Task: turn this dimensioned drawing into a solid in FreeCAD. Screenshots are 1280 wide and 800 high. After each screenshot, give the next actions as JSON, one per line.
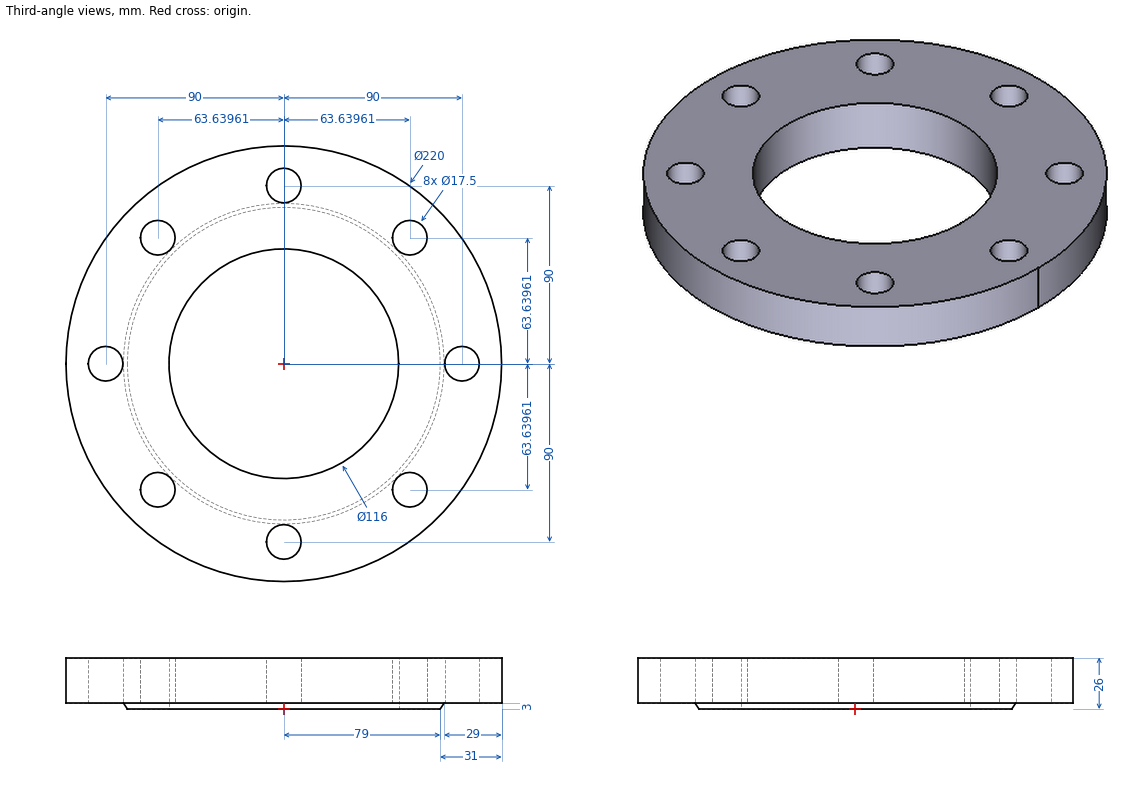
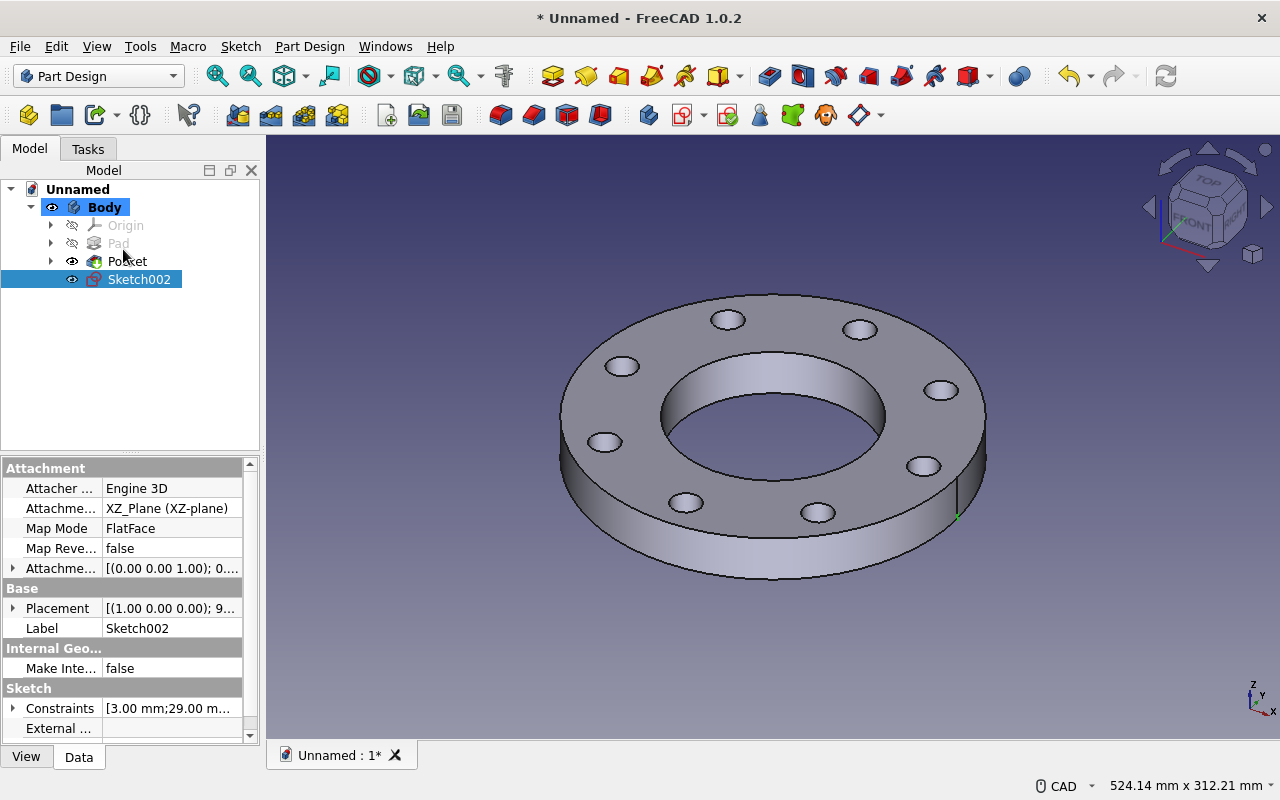
{"action": "left_click", "coordinate": [836, 76]}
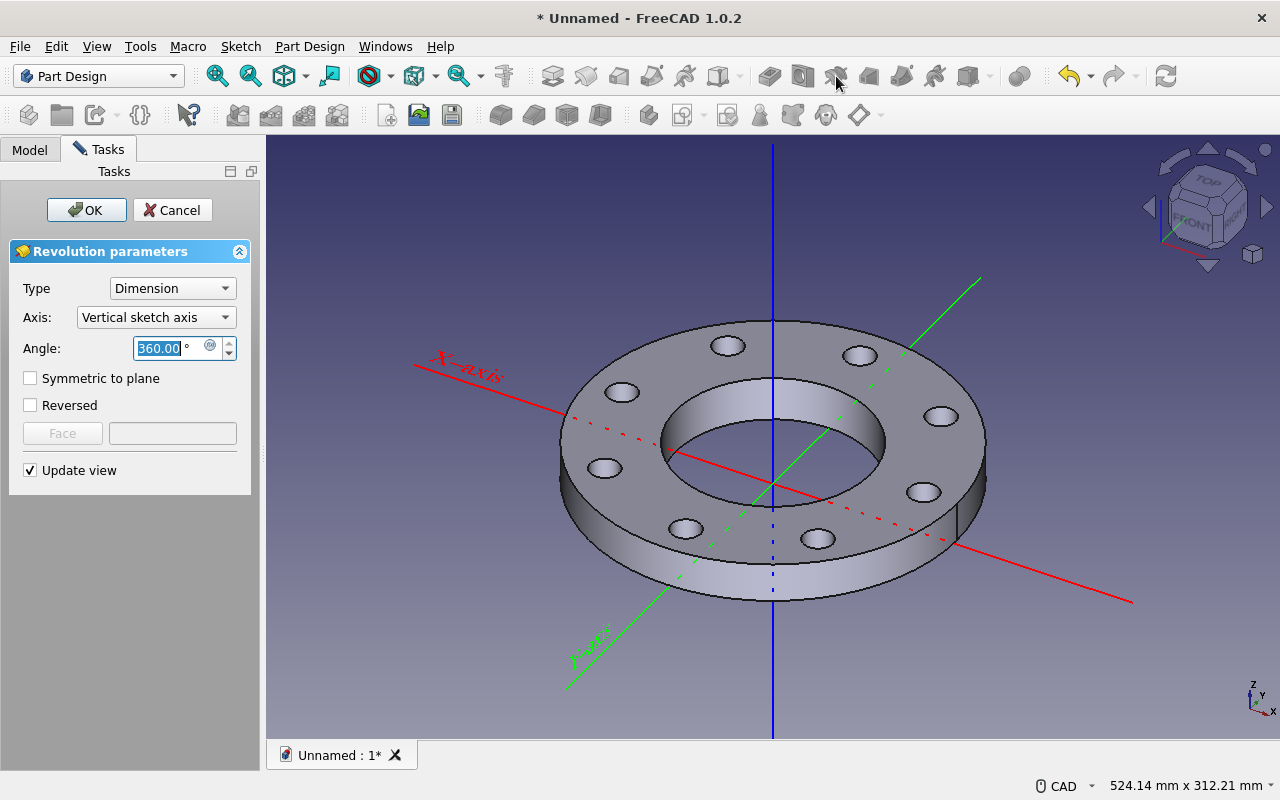
{"action": "left_click", "coordinate": [87, 210]}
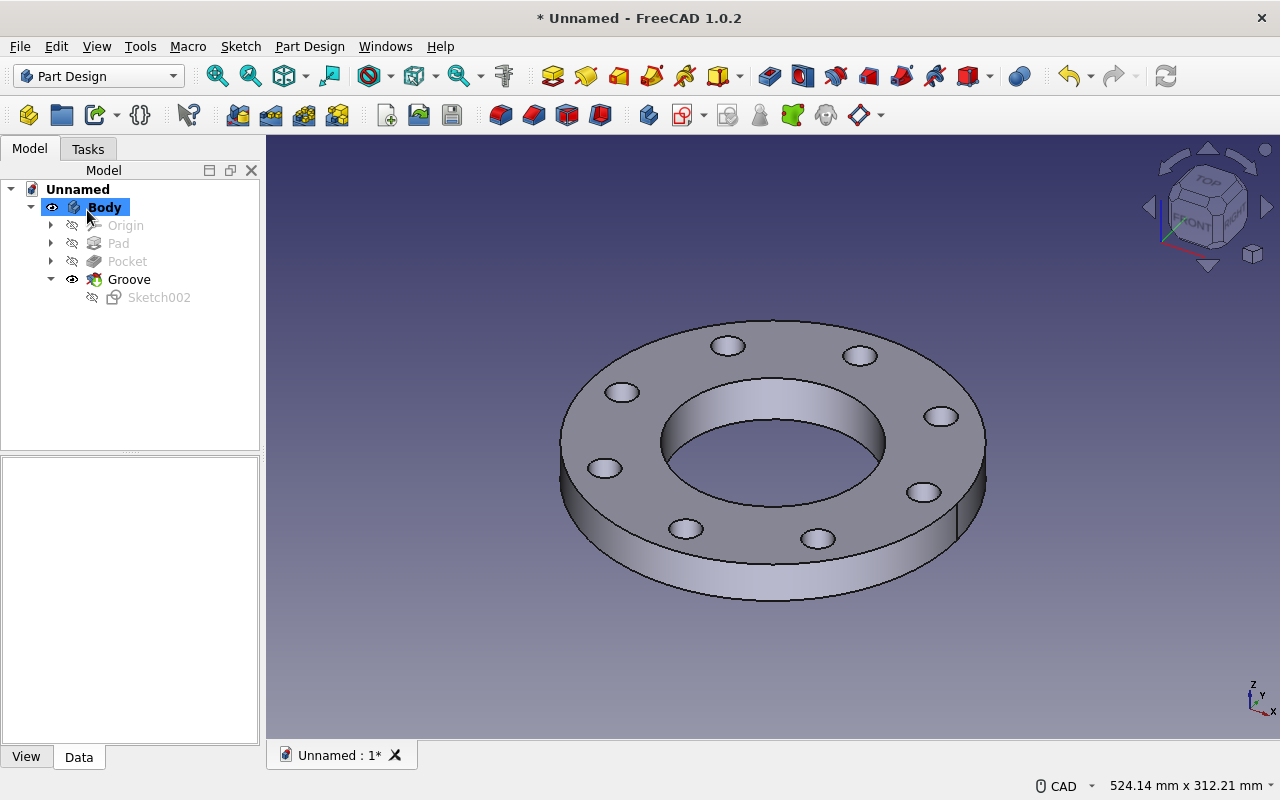
{"action": "key", "text": "0"}